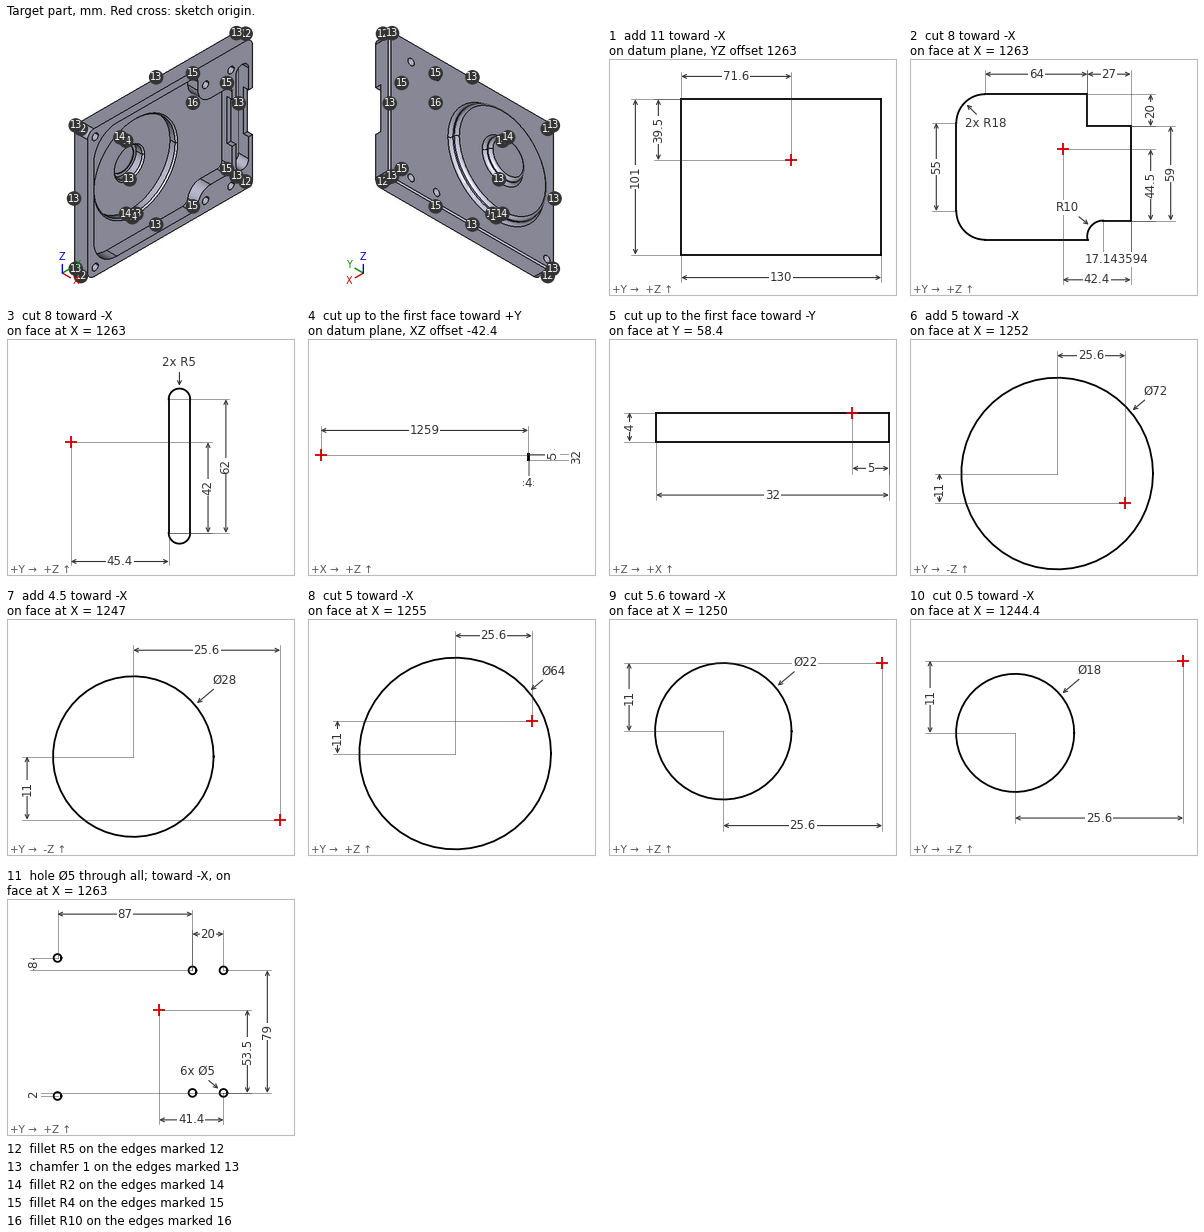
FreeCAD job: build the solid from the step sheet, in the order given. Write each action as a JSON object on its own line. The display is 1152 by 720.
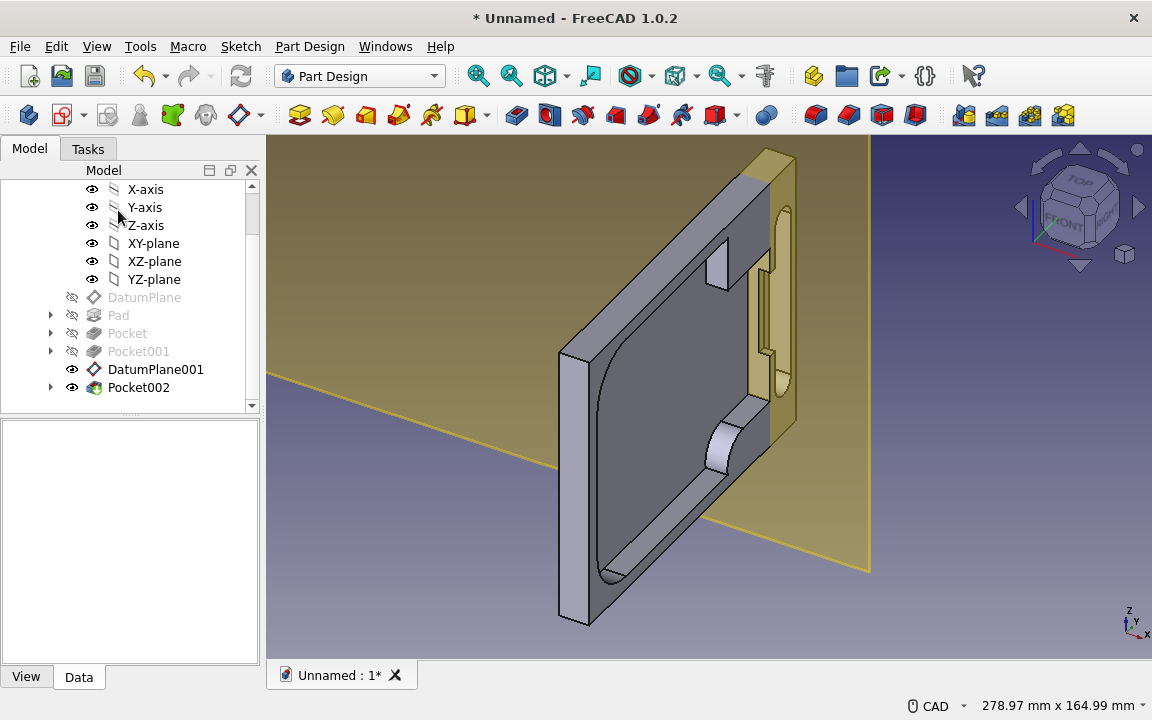
{"action": "left_click", "coordinate": [117, 369]}
{"action": "key", "text": "space"}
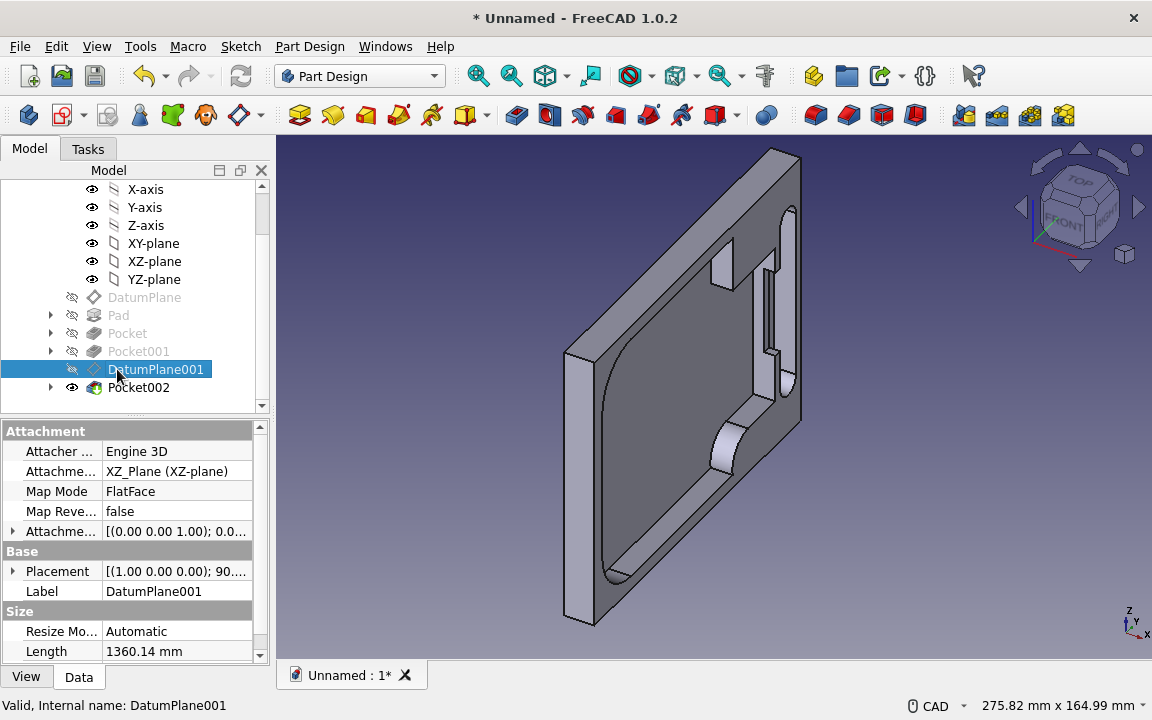
{"action": "key", "text": "4"}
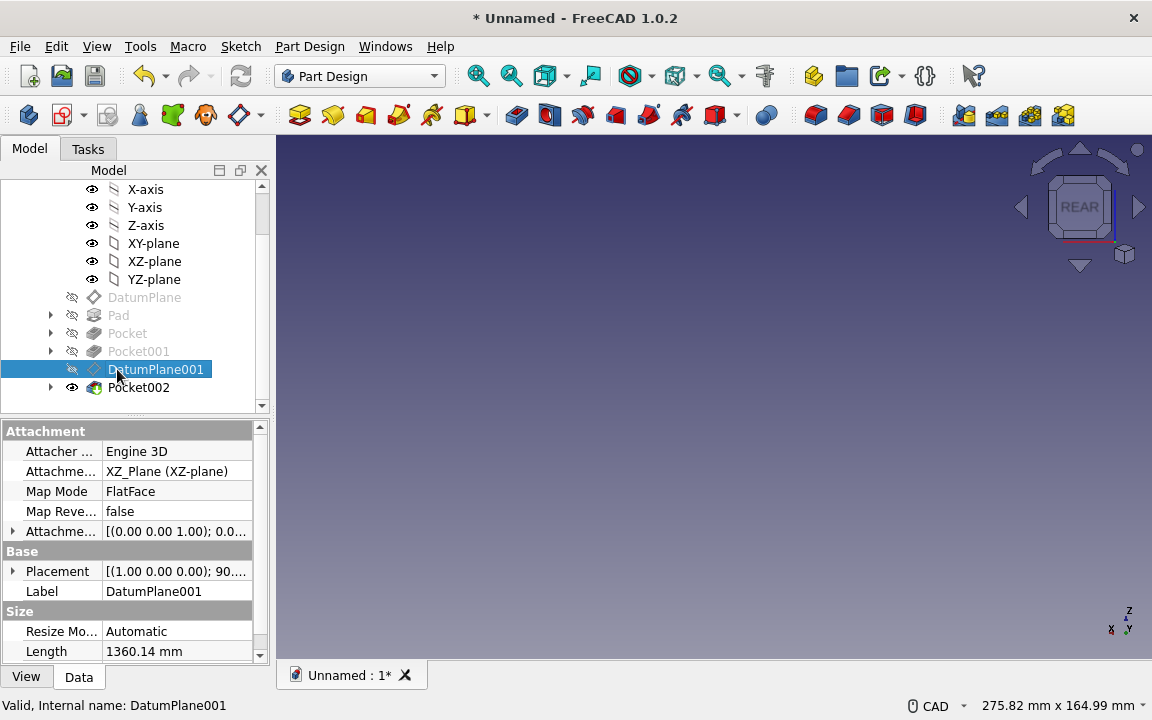
{"action": "left_click", "coordinate": [479, 76]}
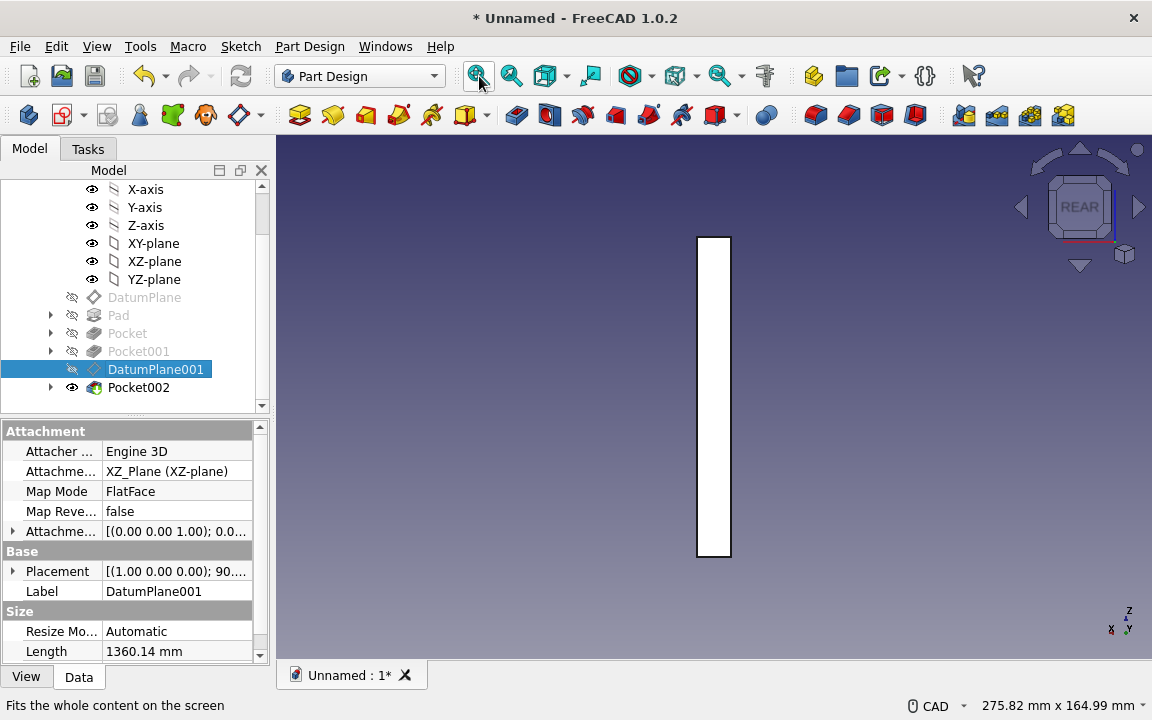
{"action": "left_click", "coordinate": [714, 259]}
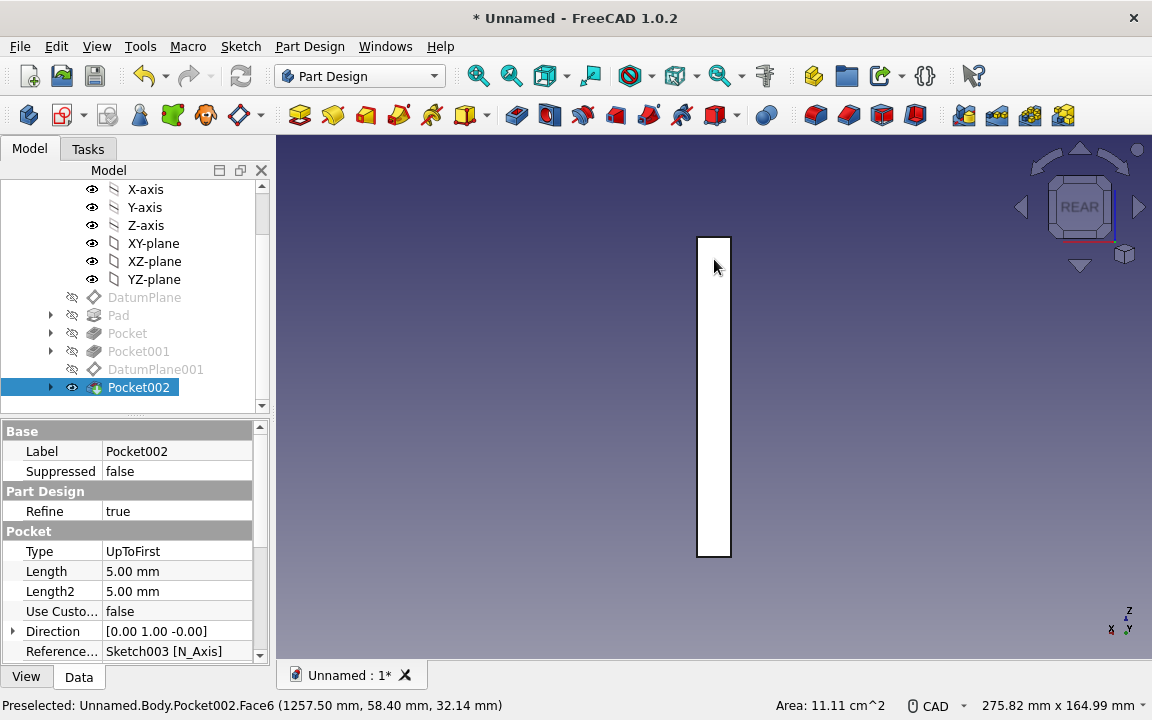
{"action": "left_click", "coordinate": [62, 116]}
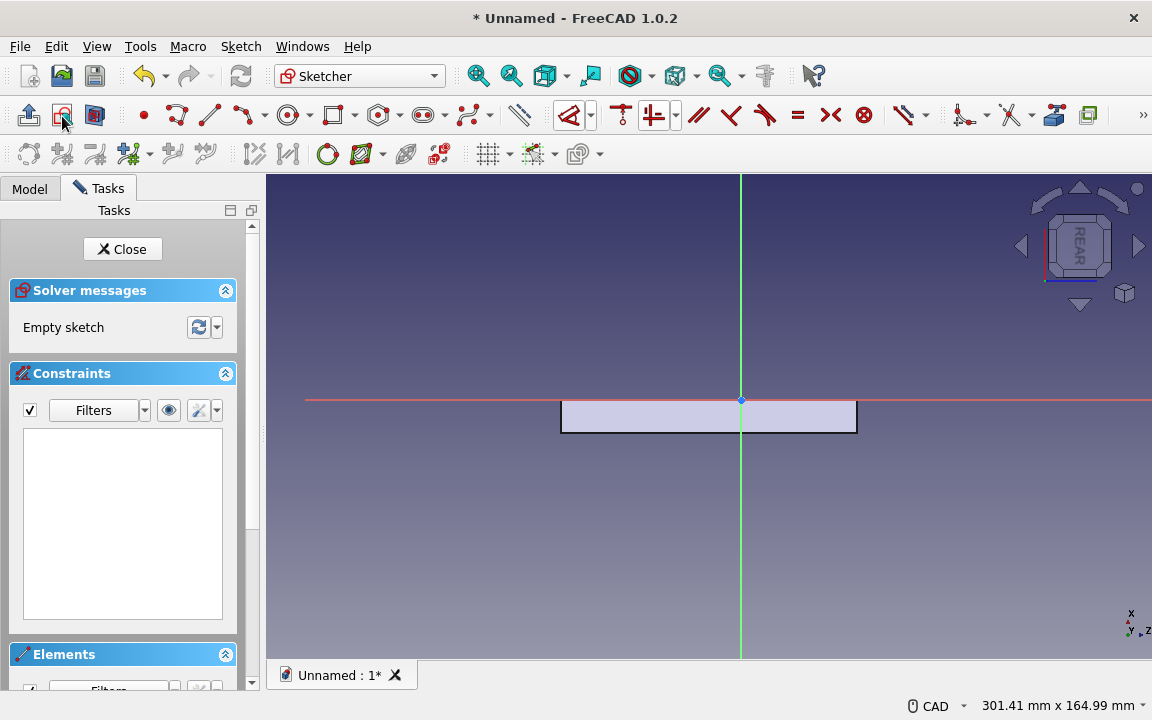
{"action": "scroll", "coordinate": [726, 404], "scroll_direction": "up", "scroll_amount": 8}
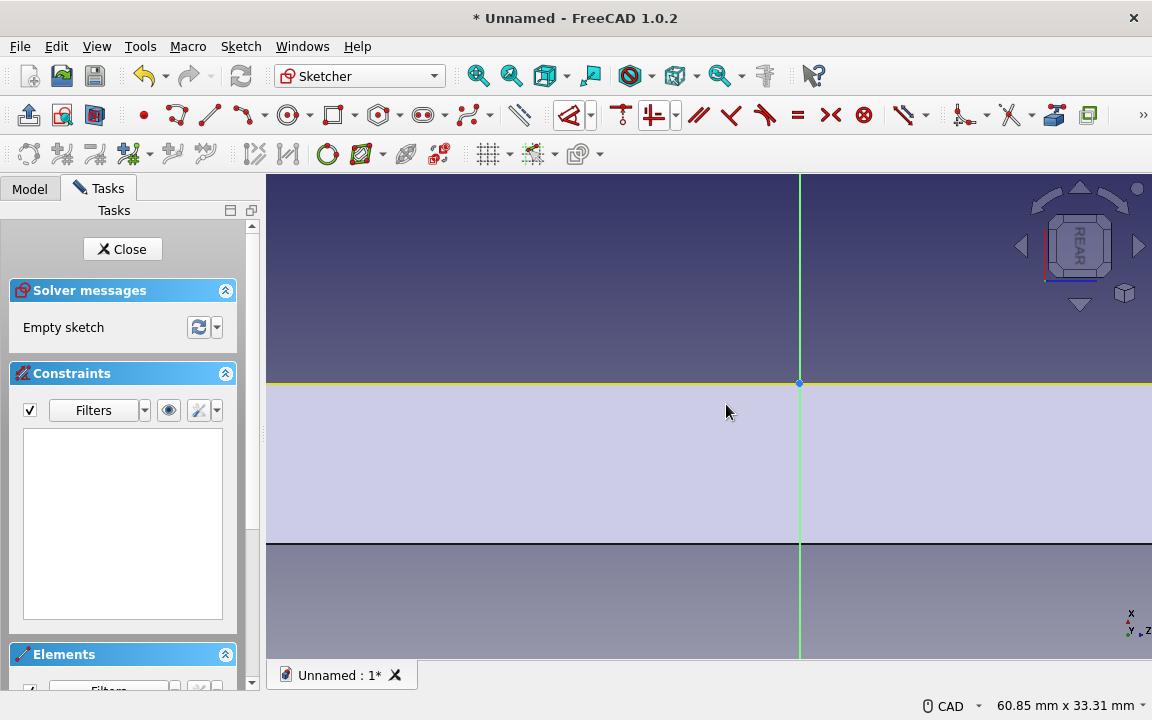
{"action": "left_click", "coordinate": [332, 116]}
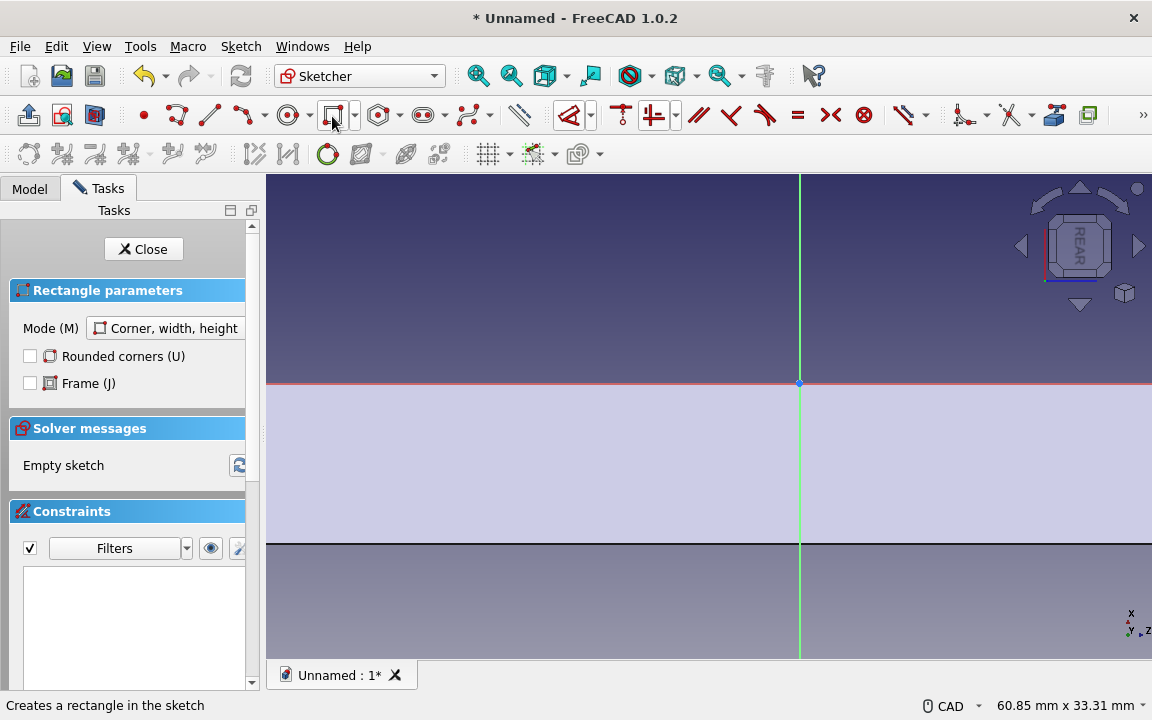
{"action": "left_click", "coordinate": [407, 384]}
{"action": "left_click", "coordinate": [873, 442]}
{"action": "key", "text": "Escape"}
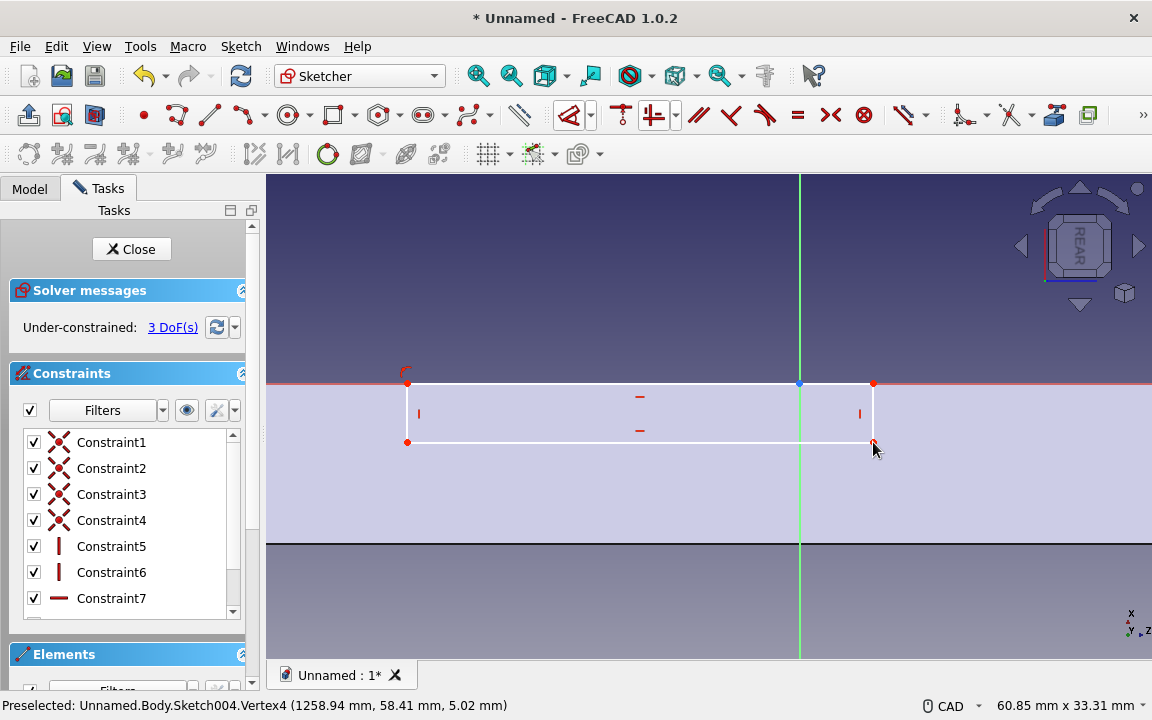
{"action": "left_click", "coordinate": [407, 402]}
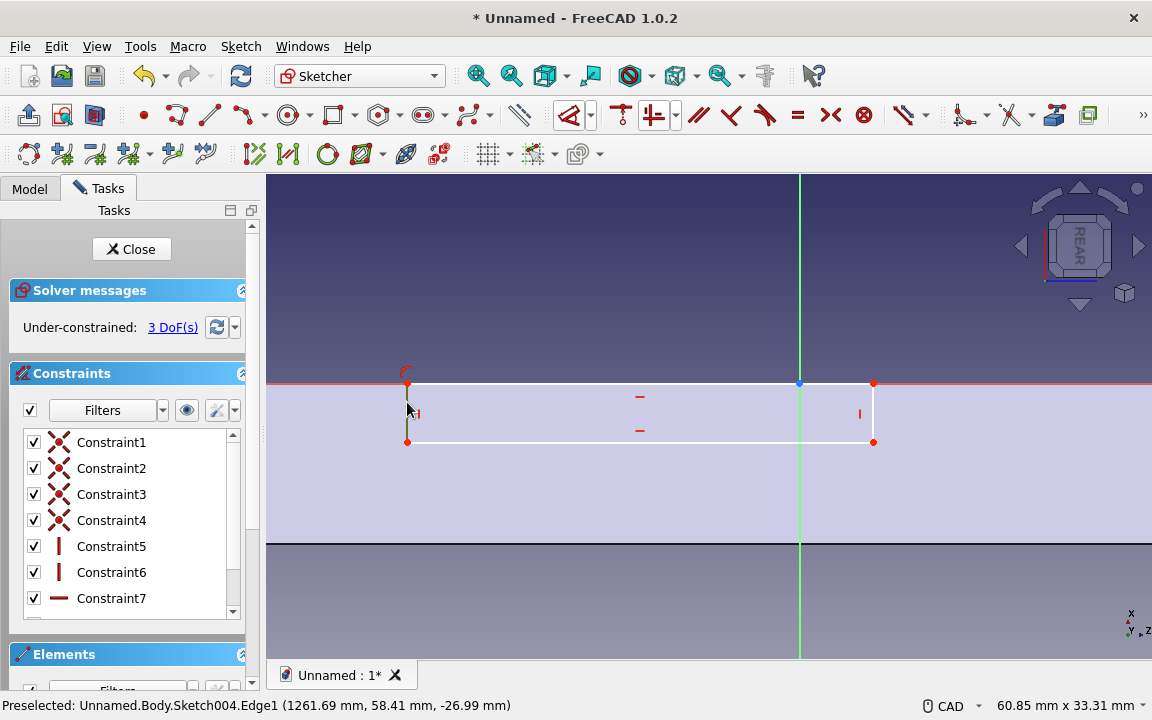
{"action": "left_click", "coordinate": [590, 116]}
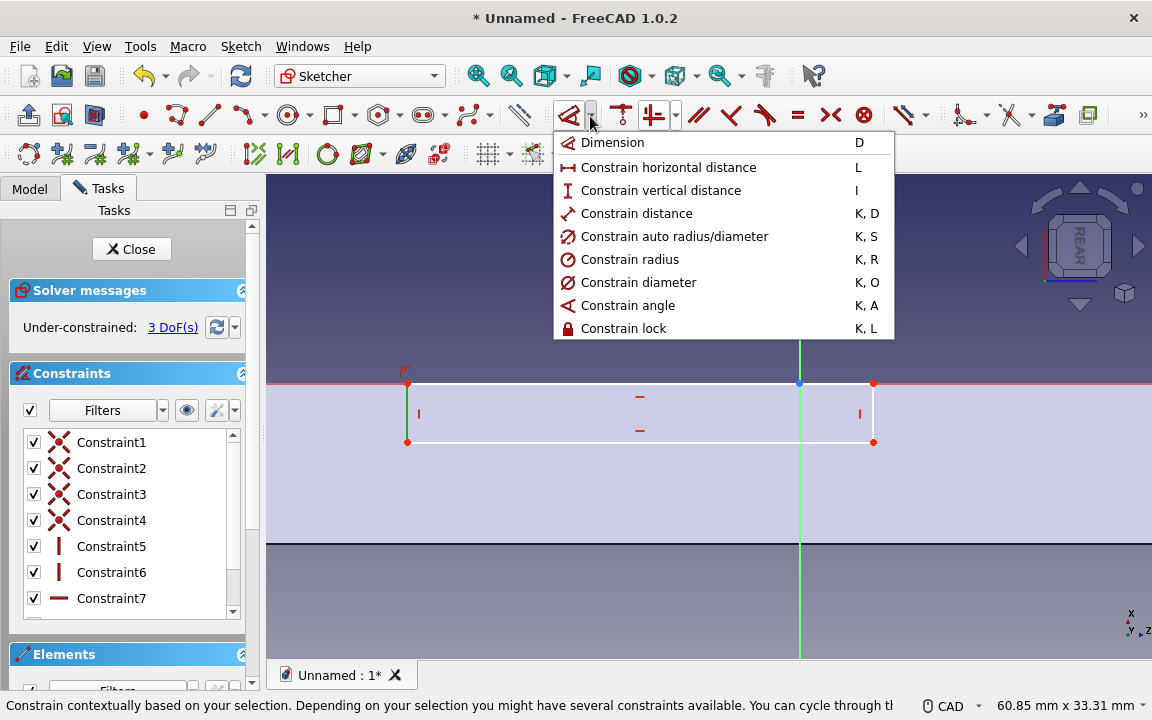
{"action": "left_click", "coordinate": [724, 190]}